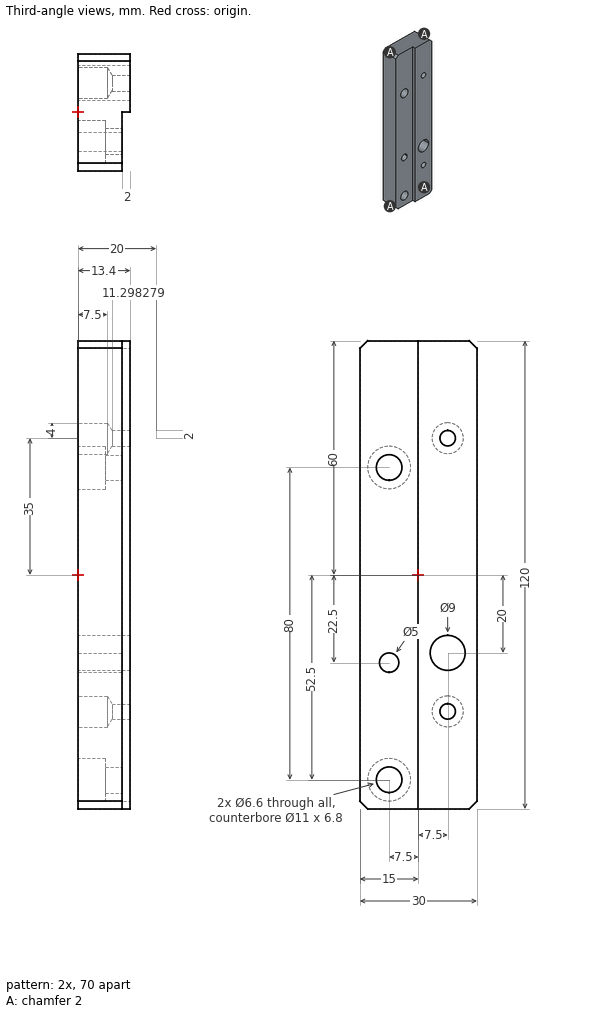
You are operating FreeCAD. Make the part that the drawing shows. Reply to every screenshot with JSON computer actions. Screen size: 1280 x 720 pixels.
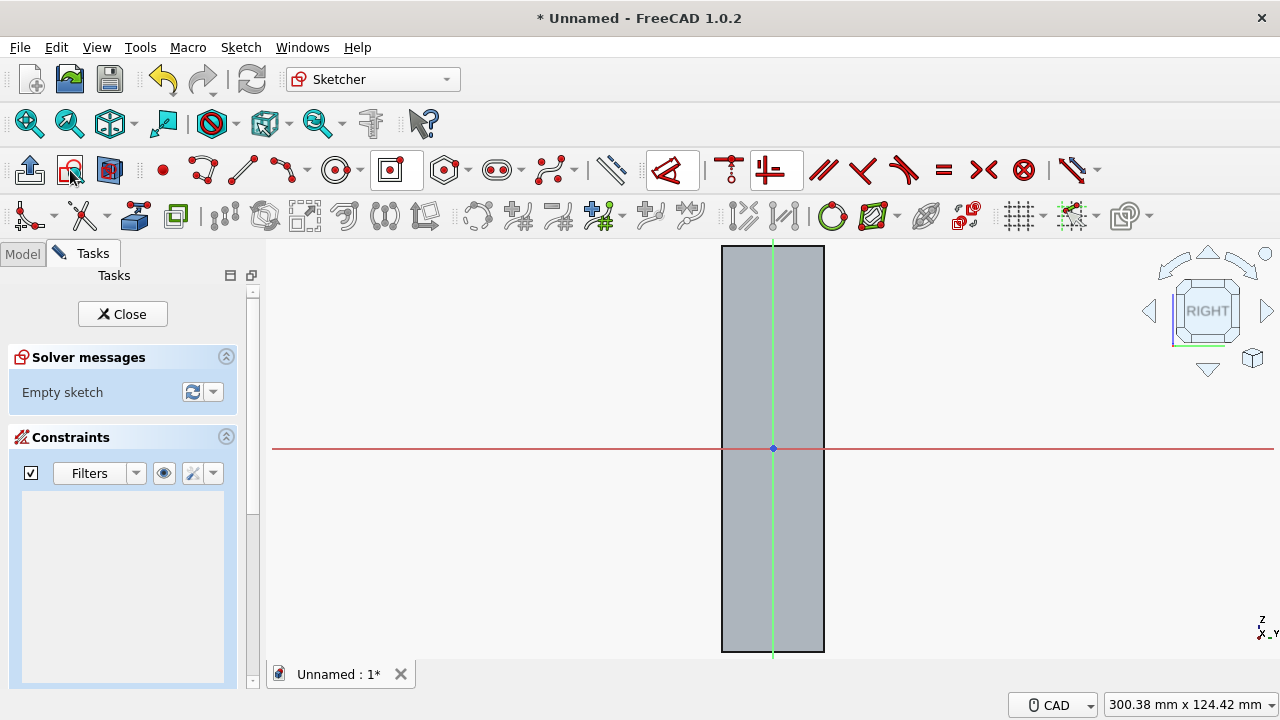
{"action": "scroll", "coordinate": [617, 449], "scroll_direction": "down", "scroll_amount": 2}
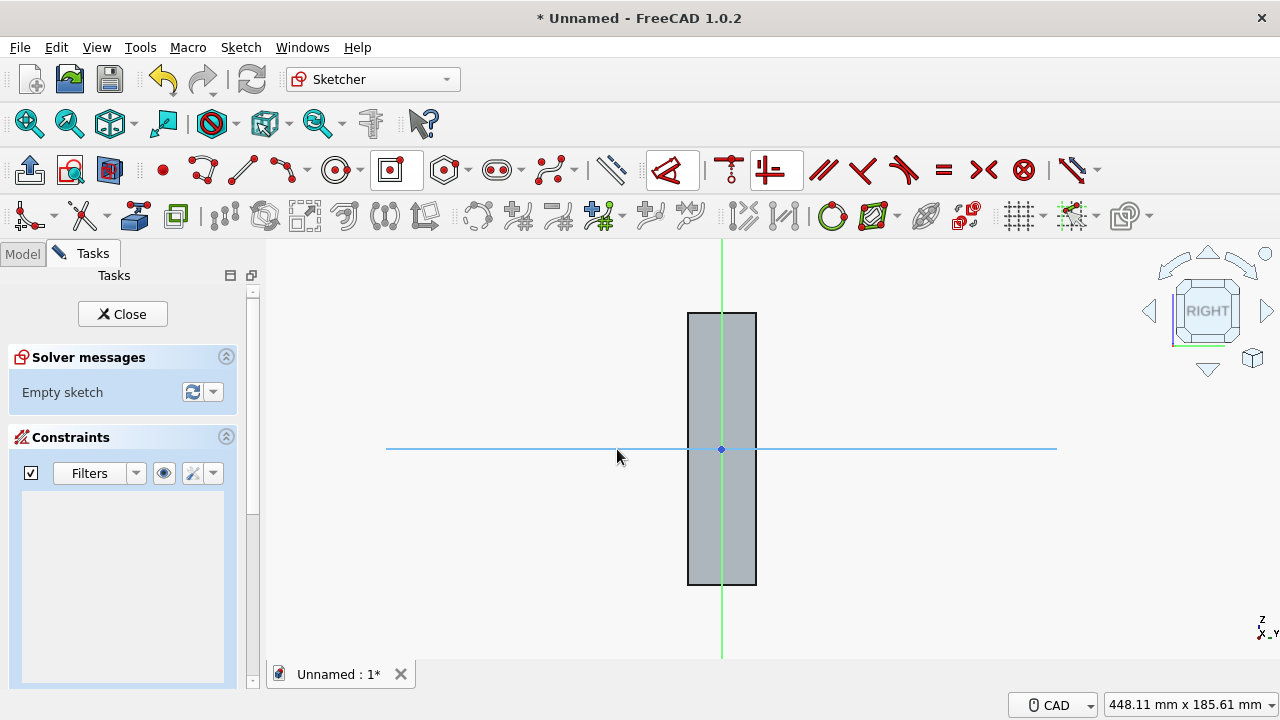
{"action": "key", "text": "g r"}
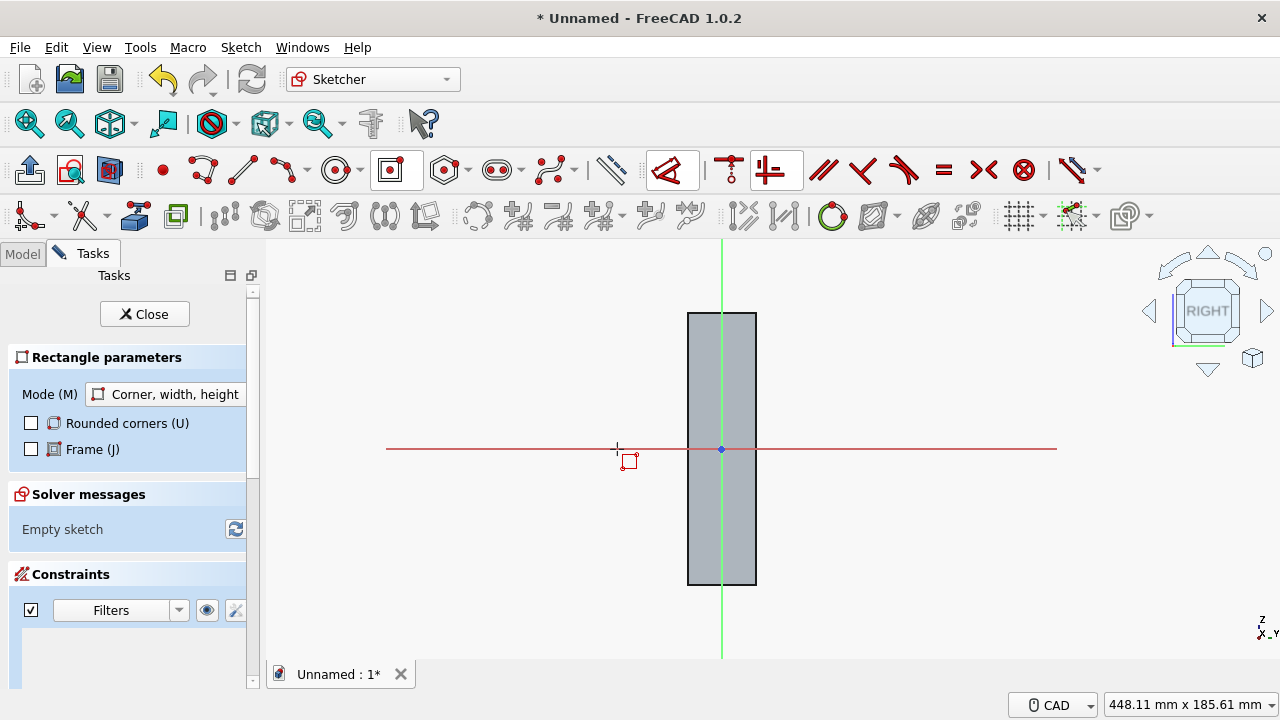
{"action": "left_click", "coordinate": [688, 313]}
{"action": "left_click", "coordinate": [722, 585]}
{"action": "key", "text": "Escape"}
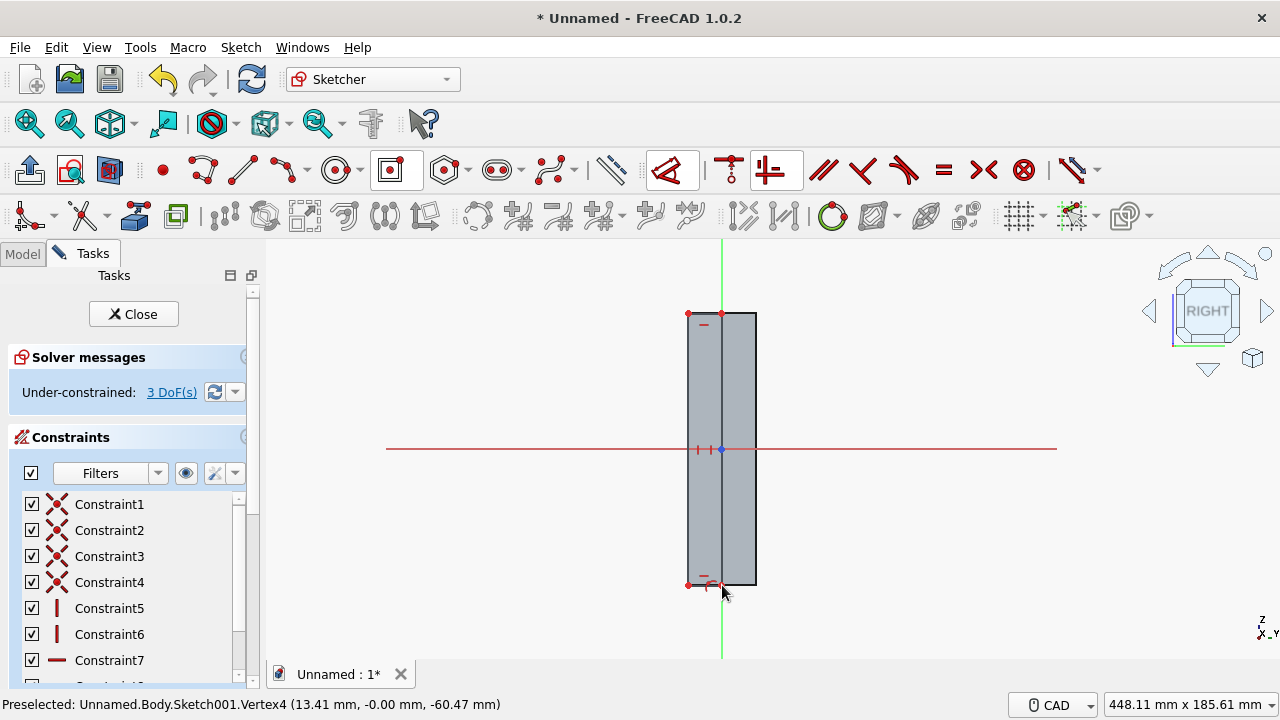
{"action": "scroll", "coordinate": [698, 586], "scroll_direction": "up", "scroll_amount": 2}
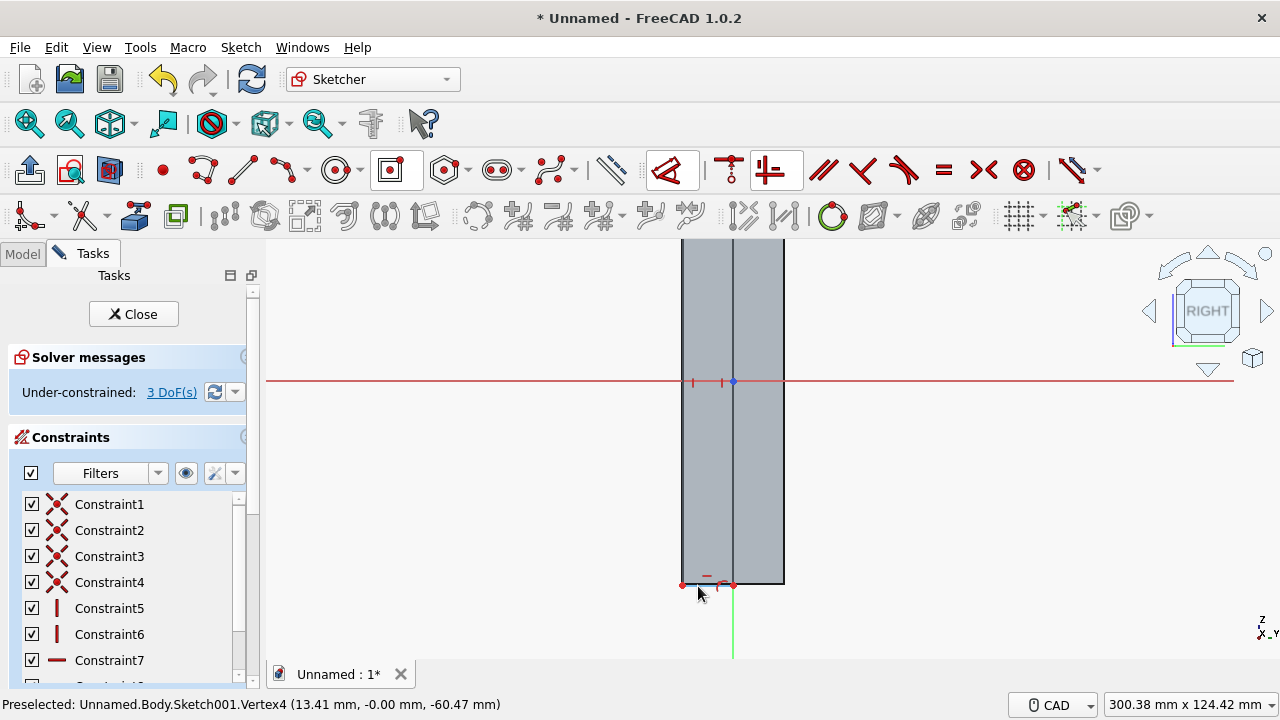
{"action": "left_click", "coordinate": [698, 586]}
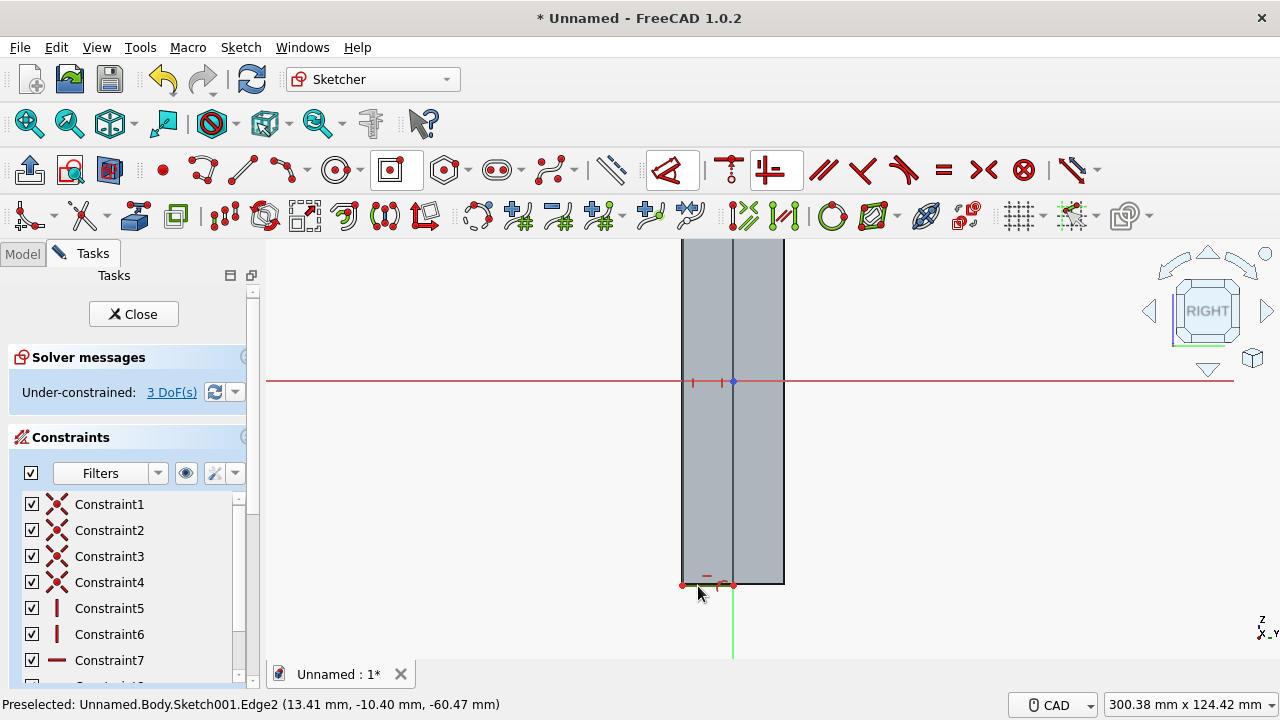
{"action": "left_click", "coordinate": [694, 170]}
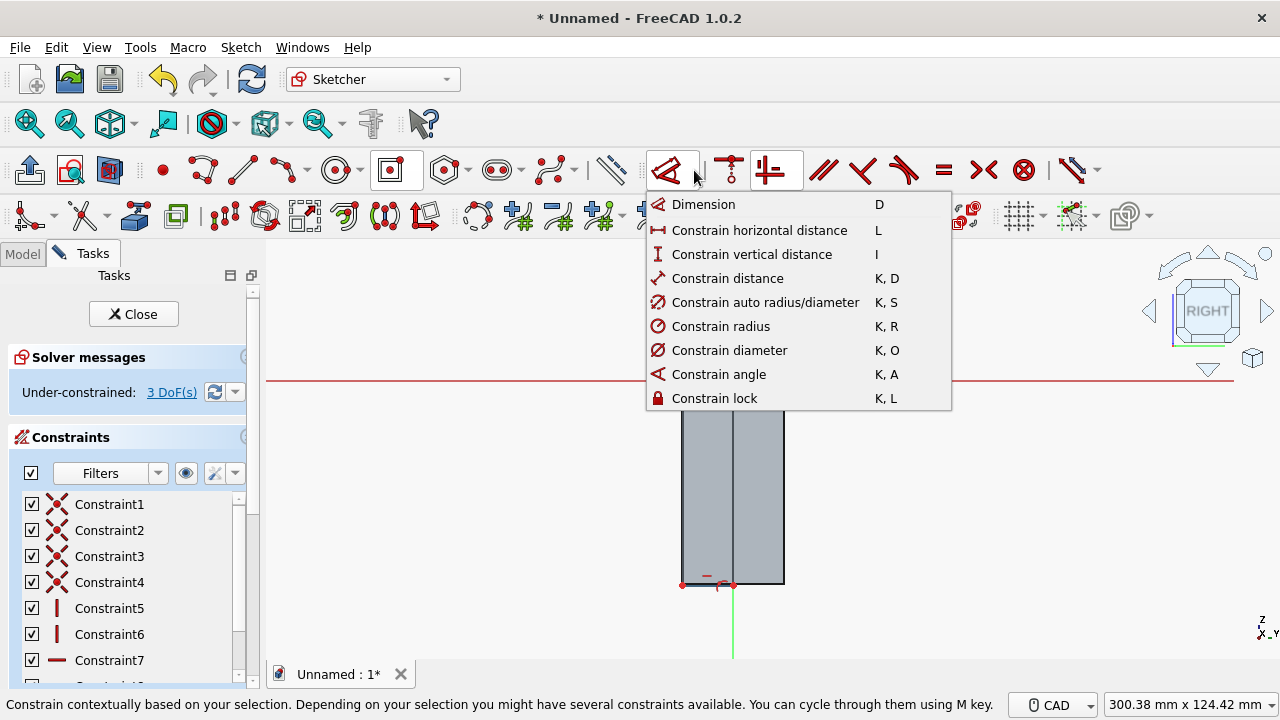
{"action": "left_click", "coordinate": [799, 230]}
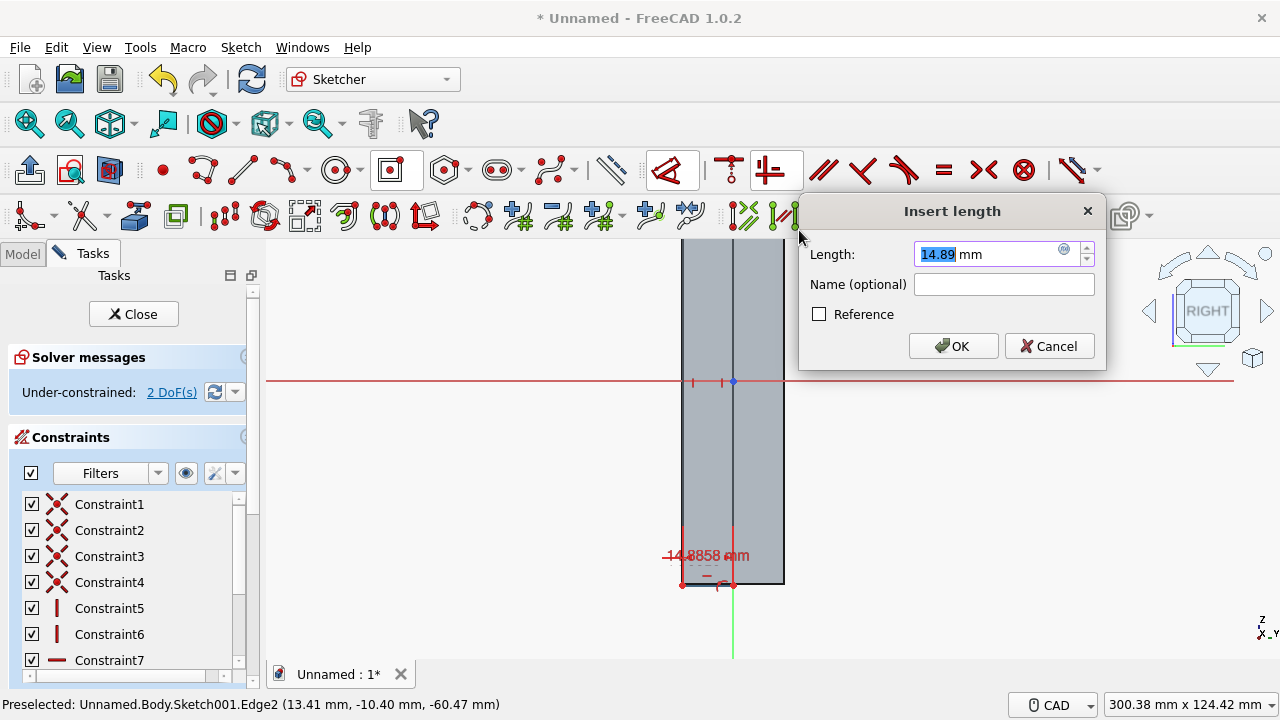
{"action": "type", "text": "15"}
{"action": "key", "text": "Return"}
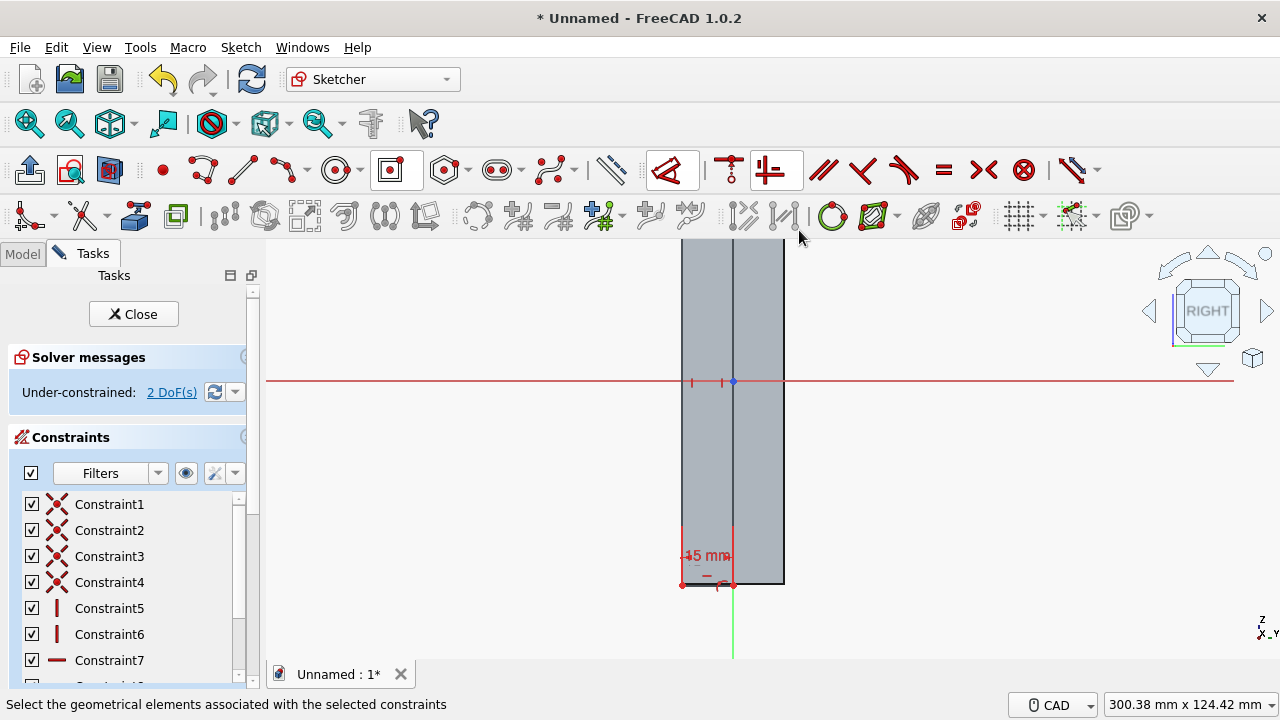
{"action": "left_click", "coordinate": [682, 302]}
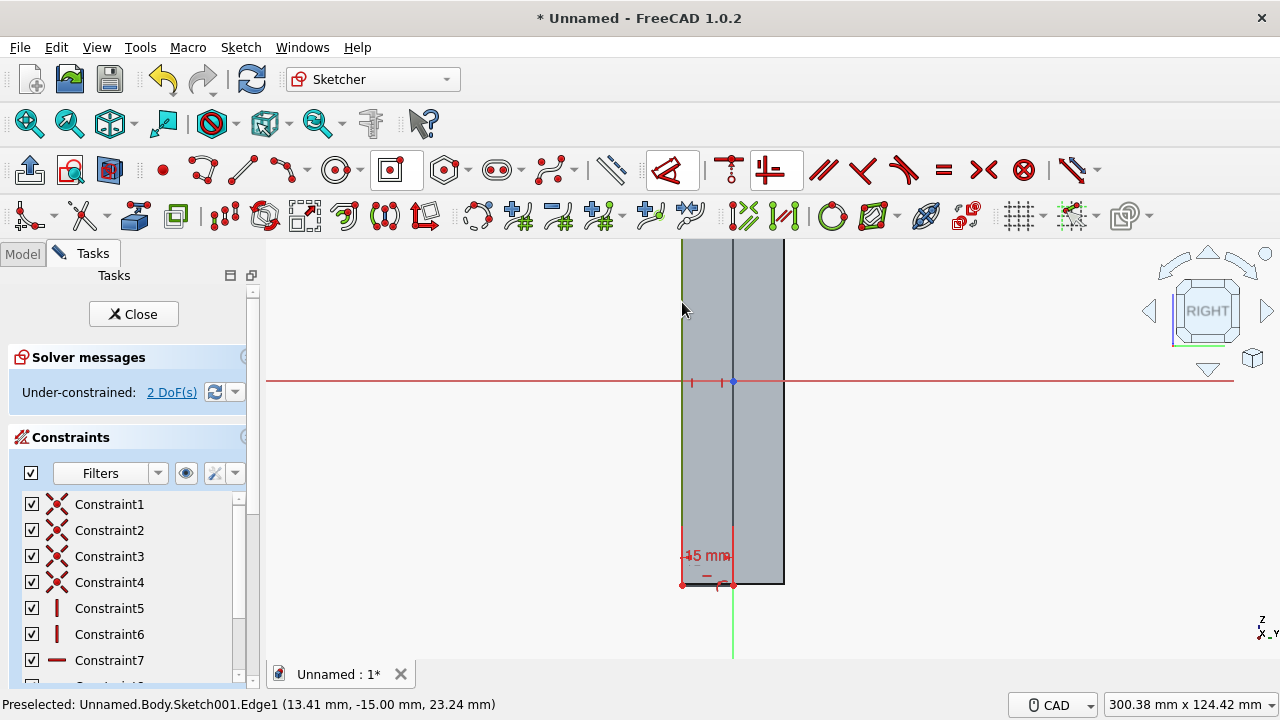
{"action": "key", "text": "i"}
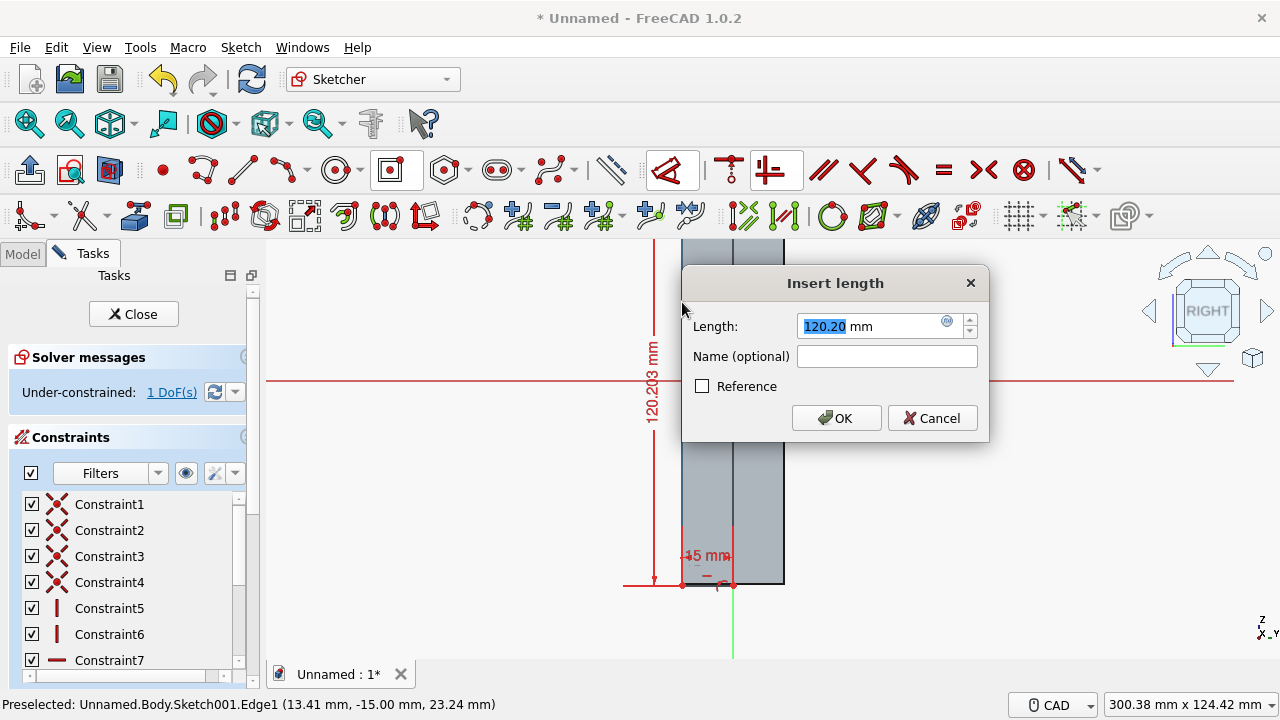
{"action": "type", "text": "120"}
{"action": "key", "text": "Return"}